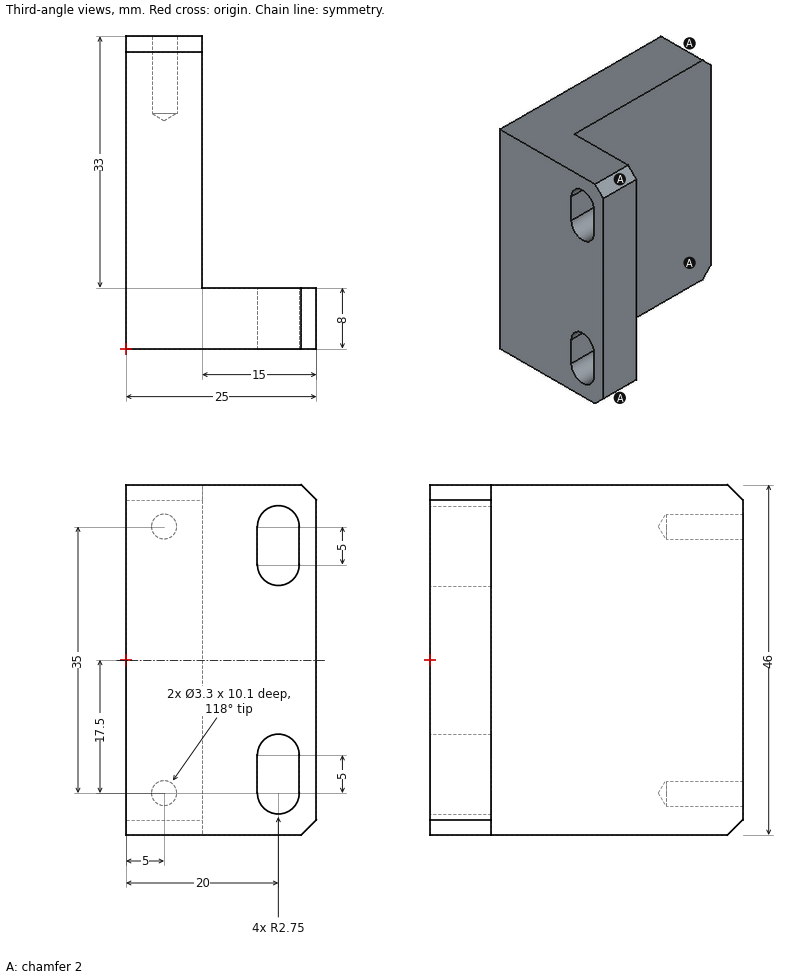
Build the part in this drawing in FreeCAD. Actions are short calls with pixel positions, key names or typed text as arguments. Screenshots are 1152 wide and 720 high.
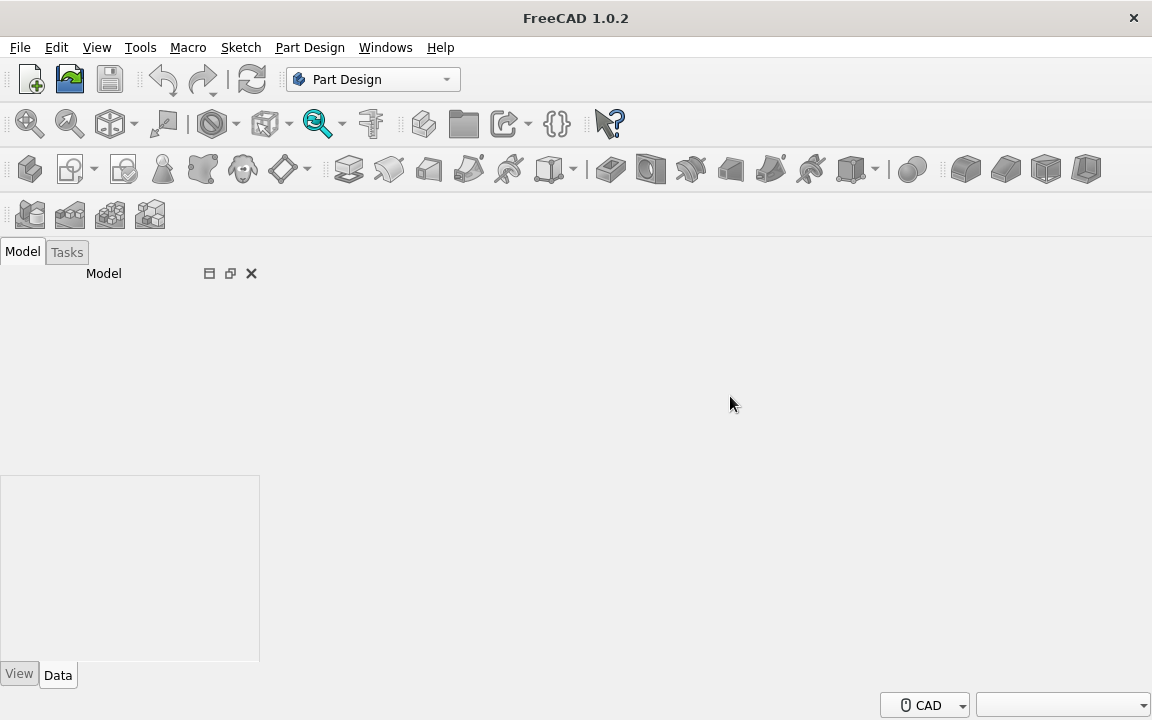
click(30, 80)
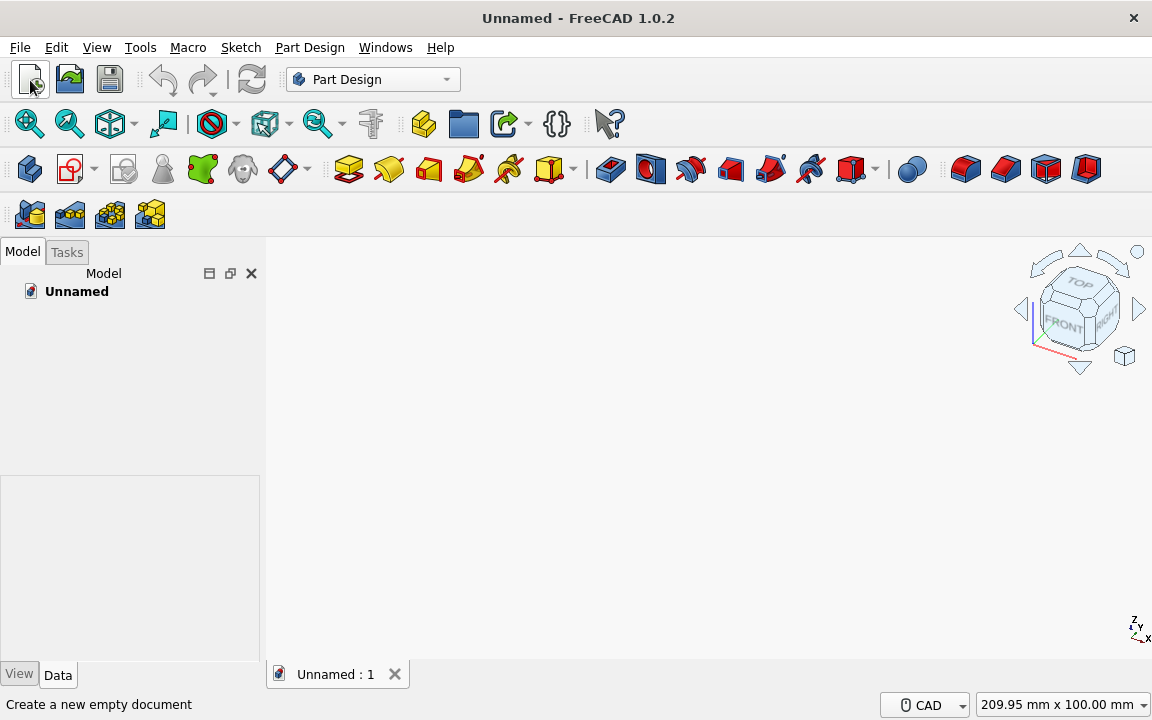
click(70, 170)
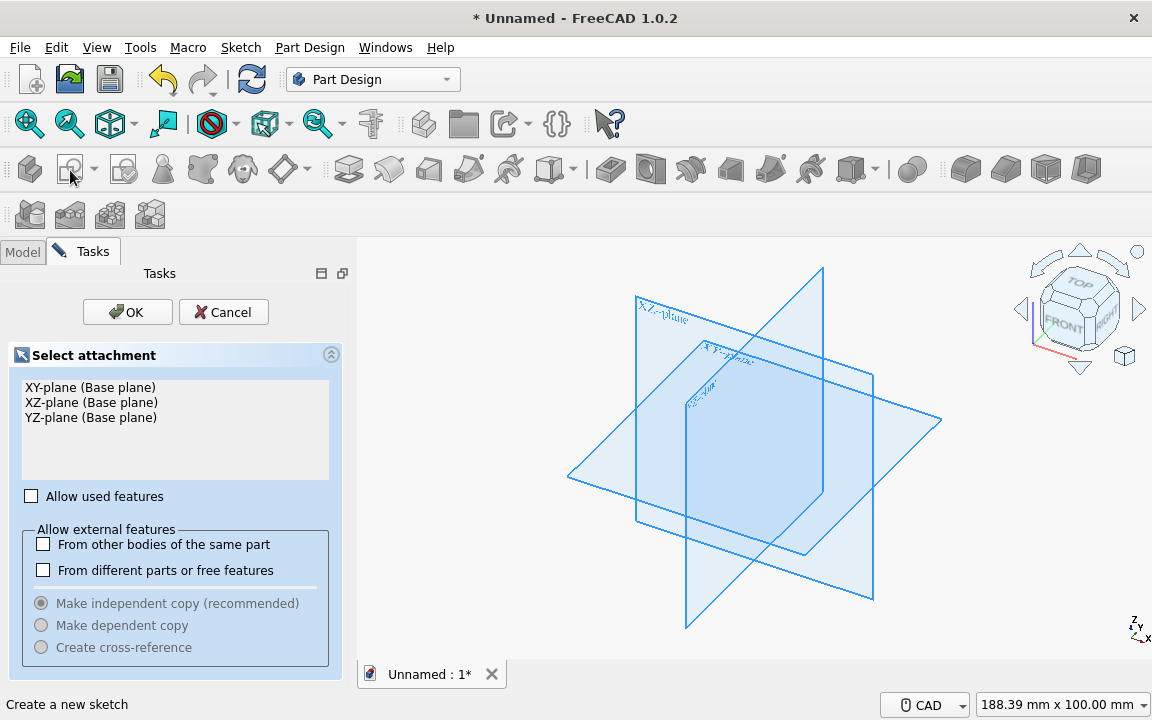
click(82, 388)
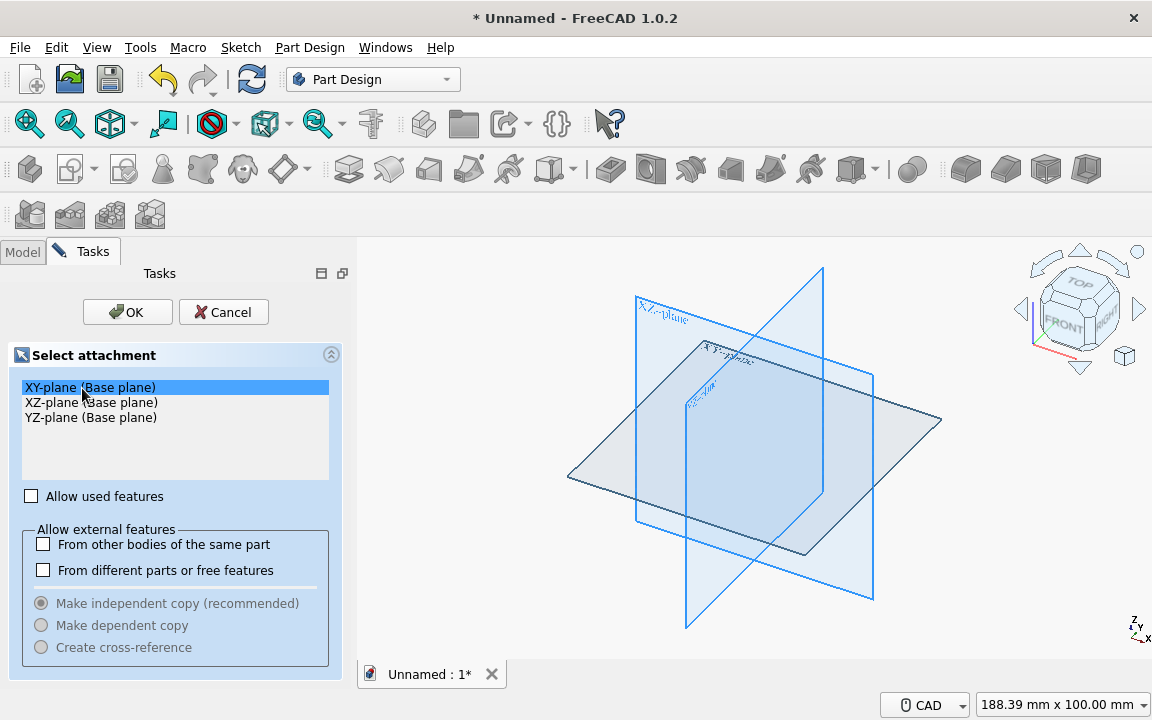
click(128, 312)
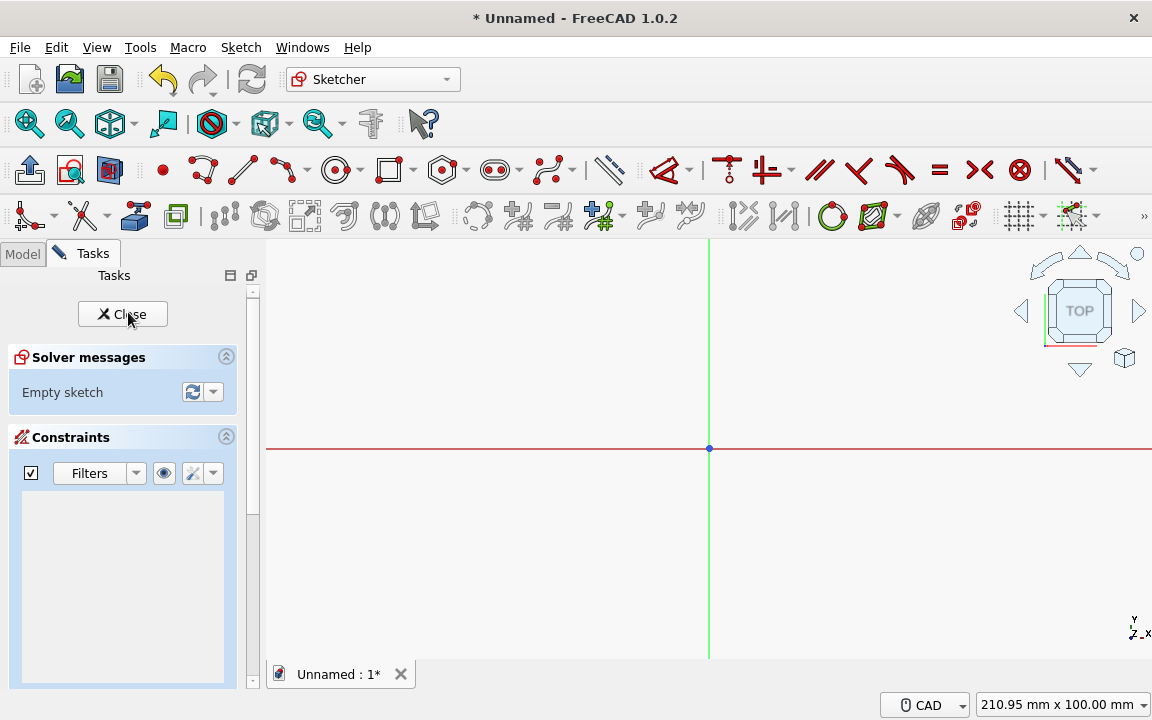
scroll(294, 631, down, 1)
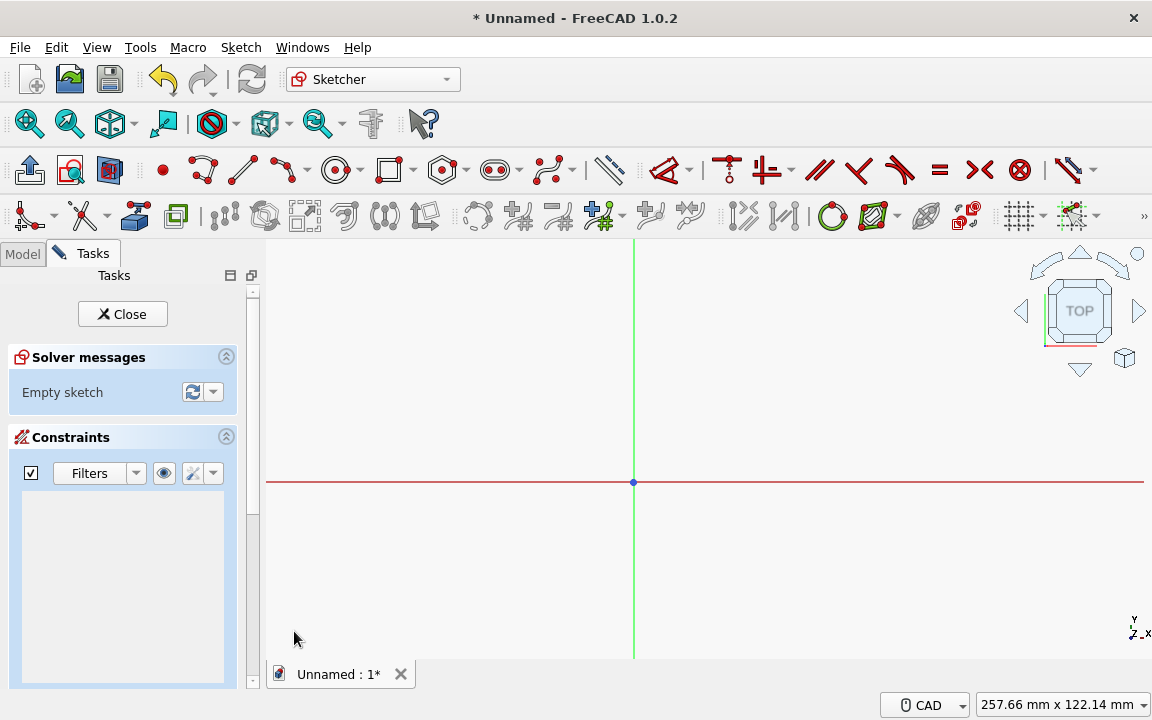
scroll(721, 366, up, 3)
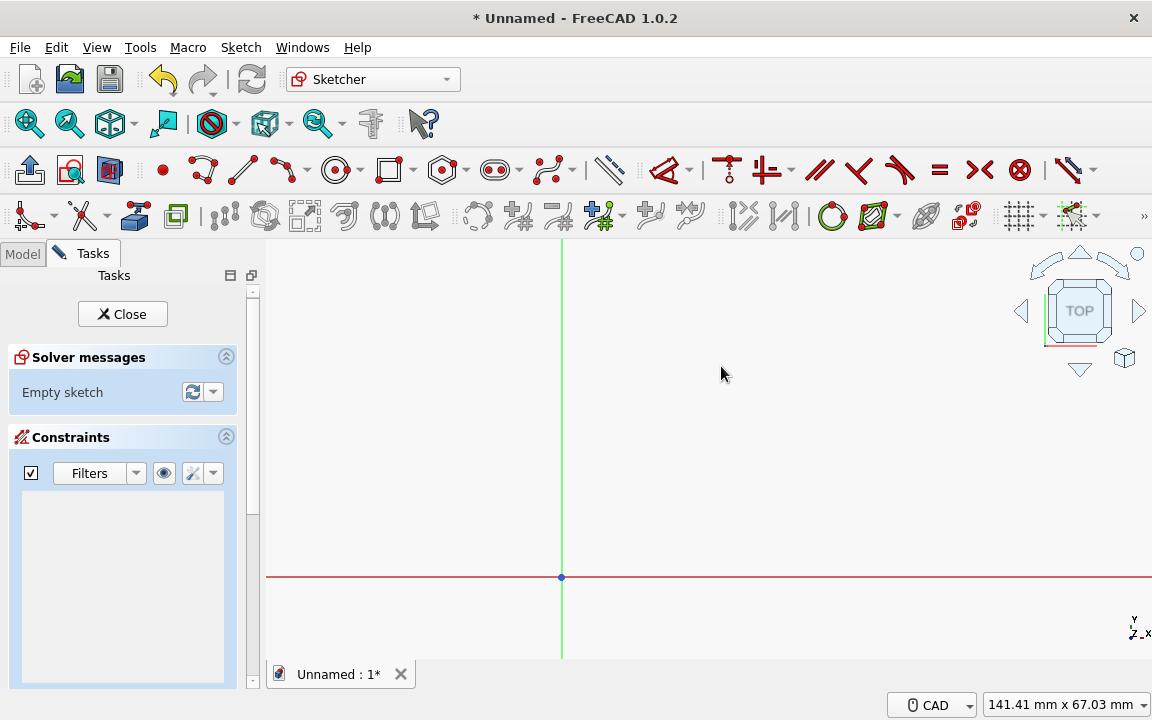
key(g)
key(m)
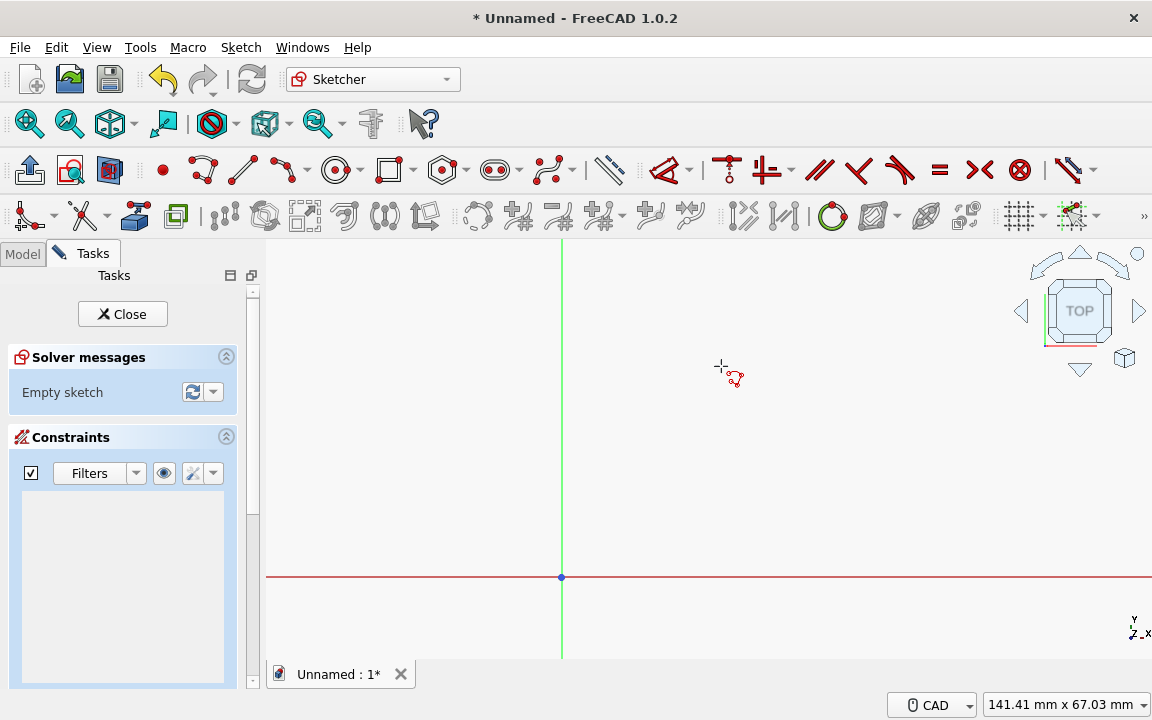
click(562, 577)
click(718, 568)
click(718, 527)
click(624, 527)
click(624, 321)
click(571, 321)
click(562, 577)
key(Escape)
key(Escape)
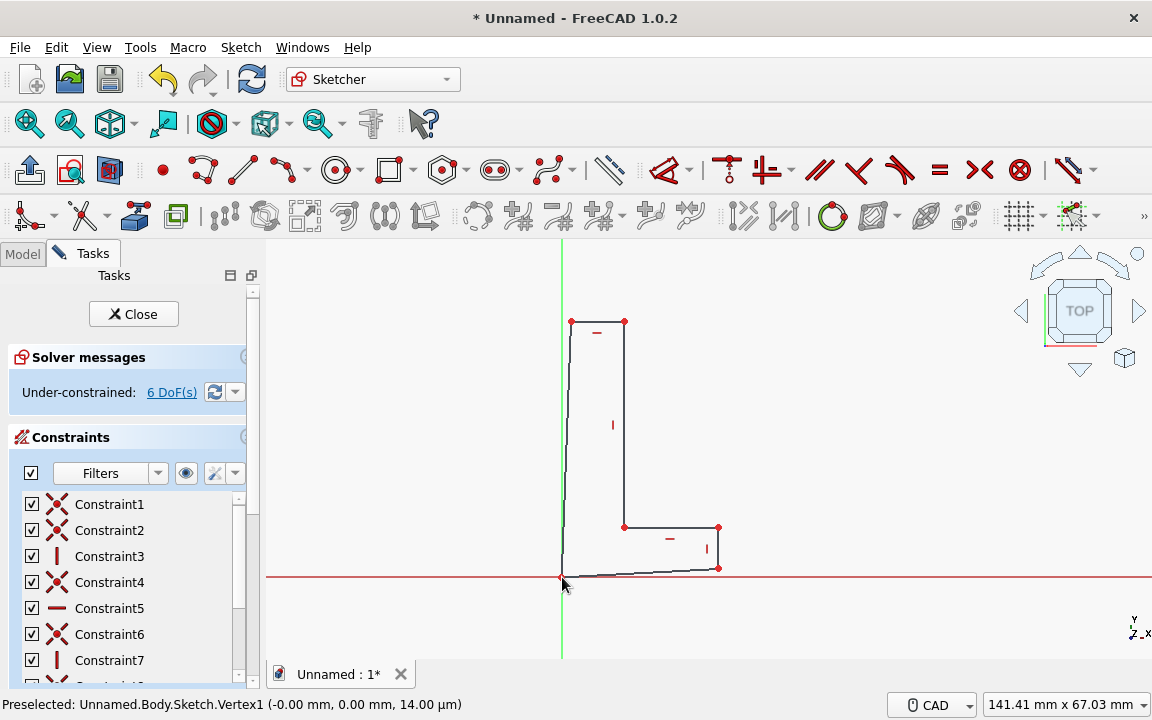
click(609, 575)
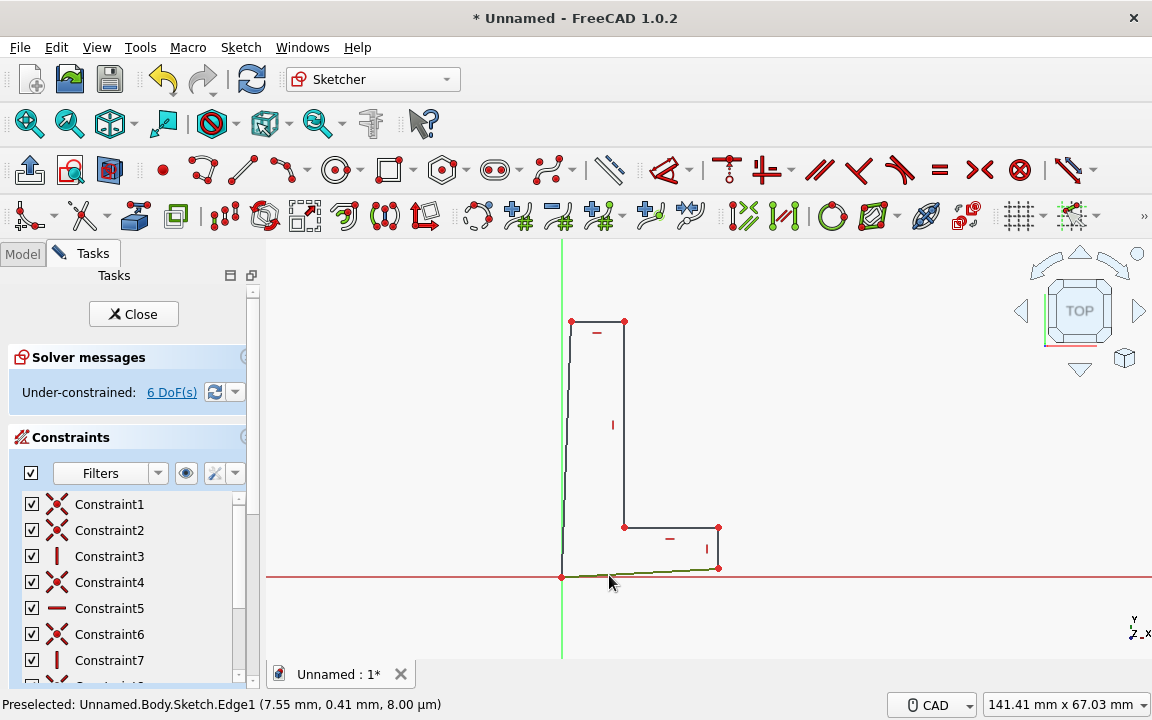
click(794, 170)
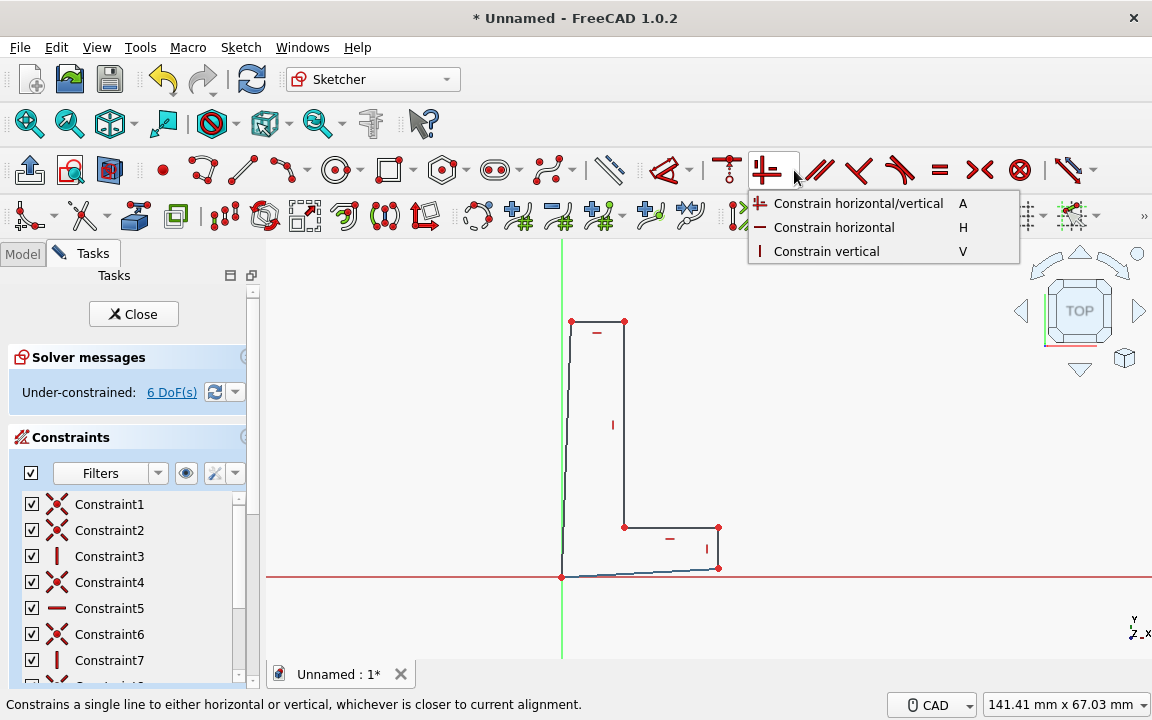
click(884, 227)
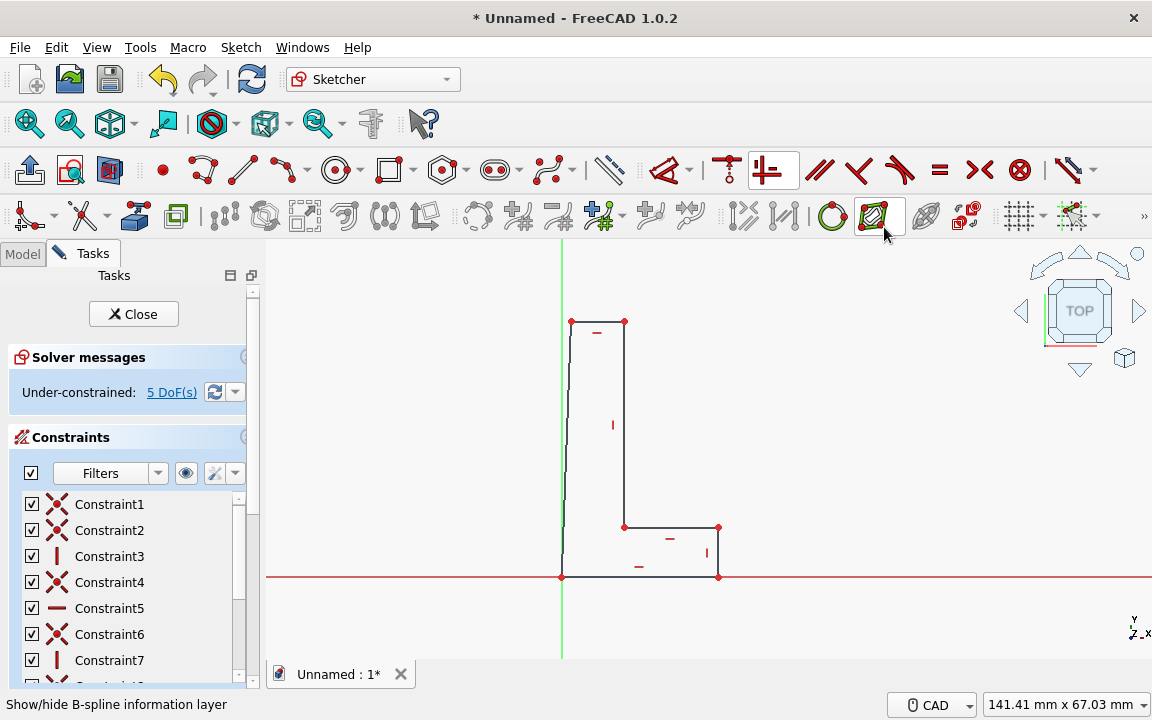
click(564, 501)